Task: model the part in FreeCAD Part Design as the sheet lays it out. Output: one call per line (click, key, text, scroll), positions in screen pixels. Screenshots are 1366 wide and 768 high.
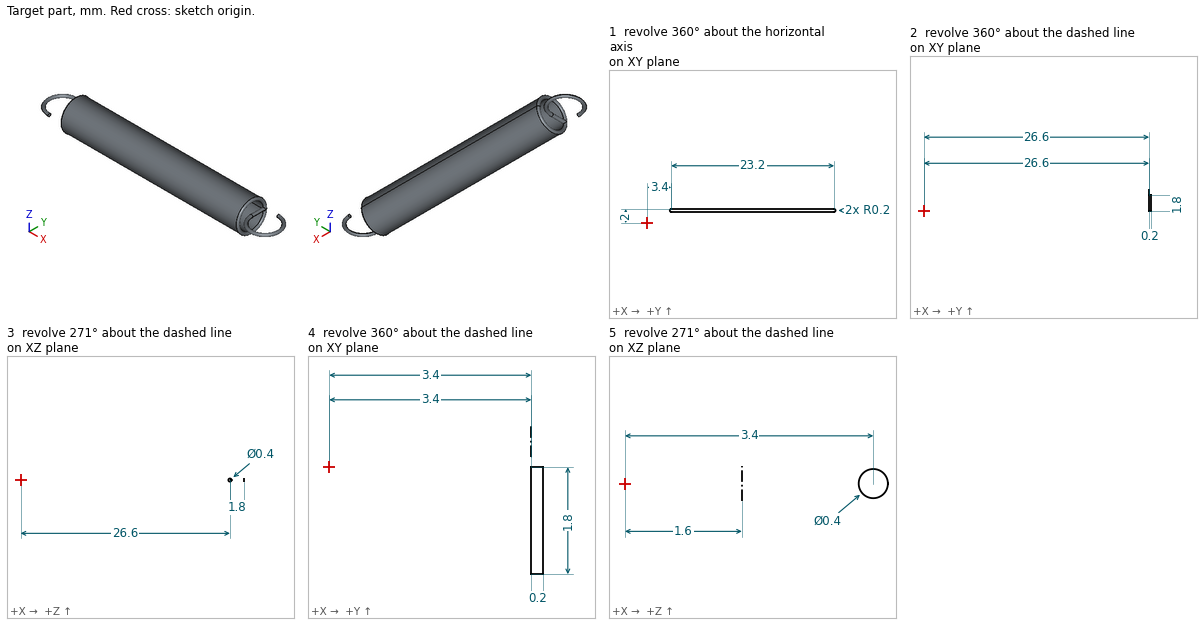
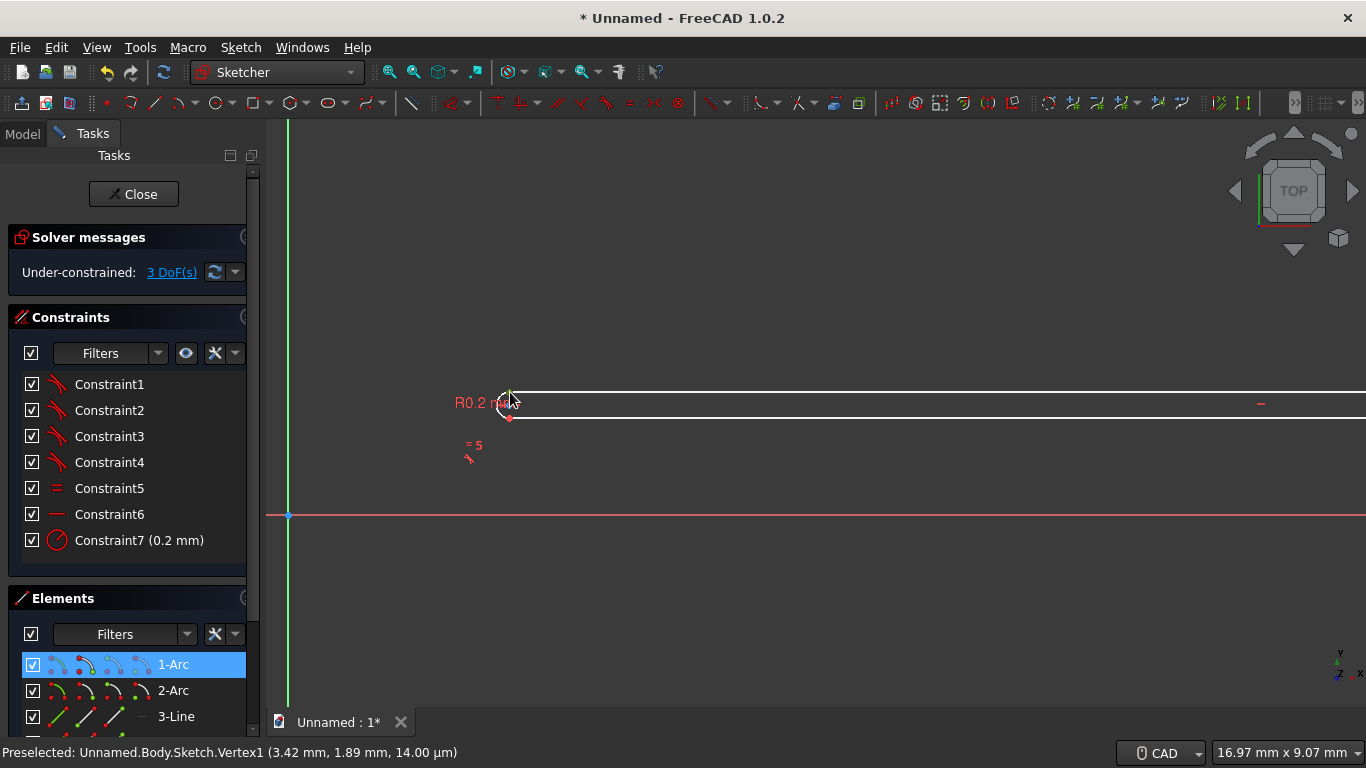
click(470, 104)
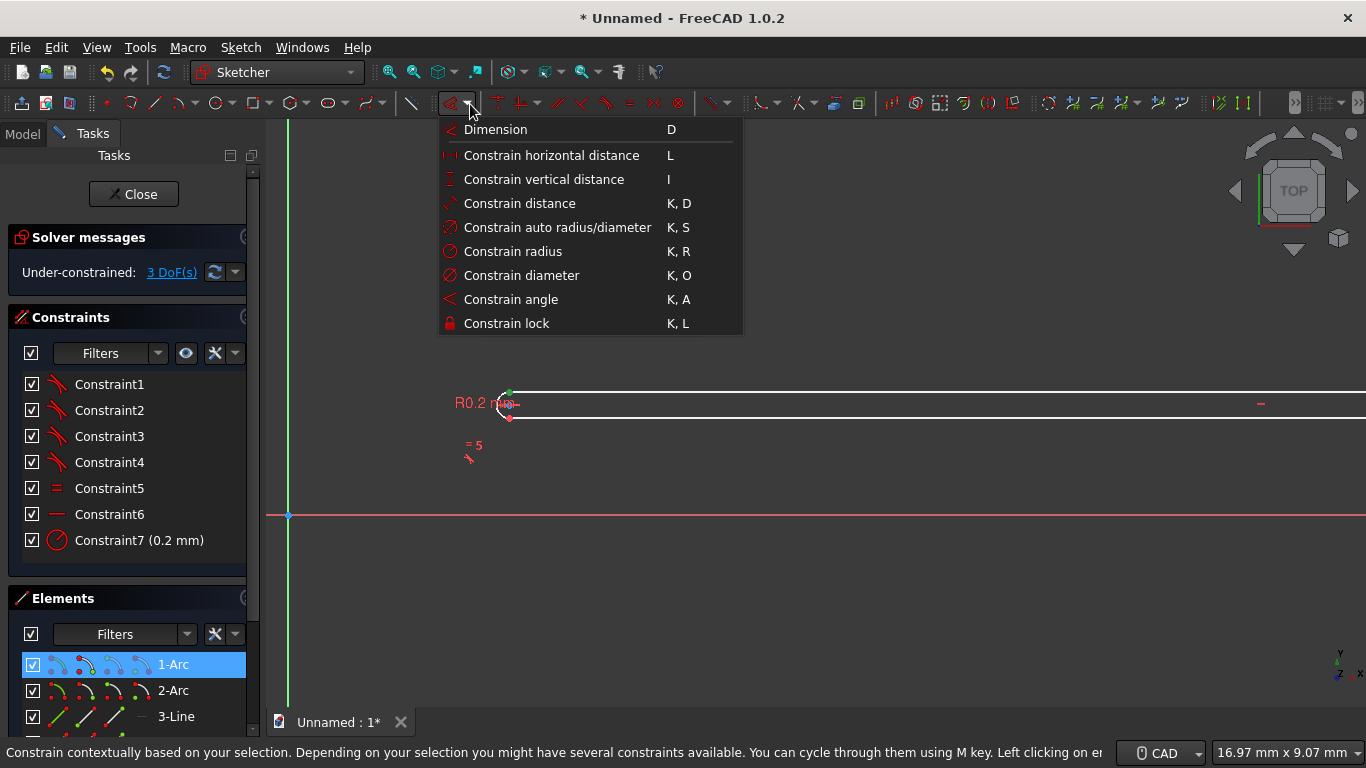
click(591, 179)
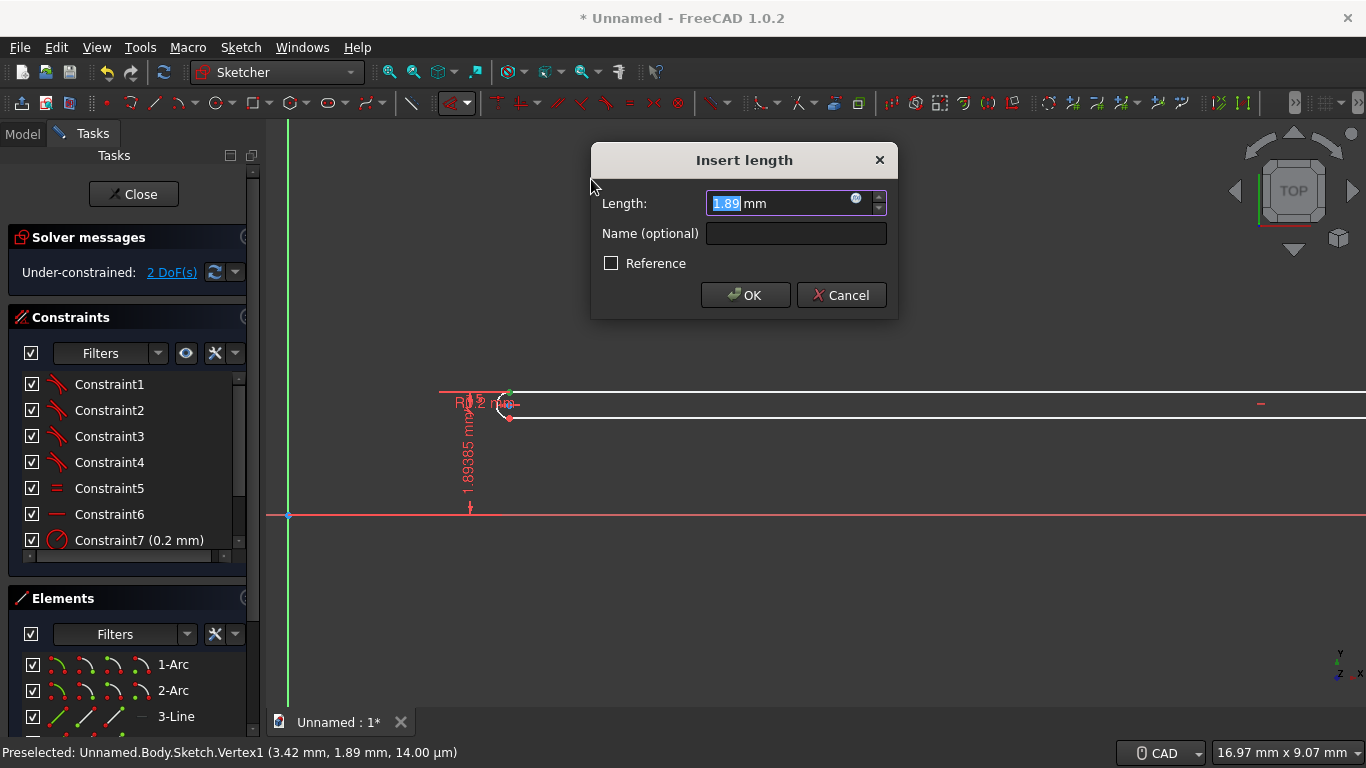
text(2)
key(Return)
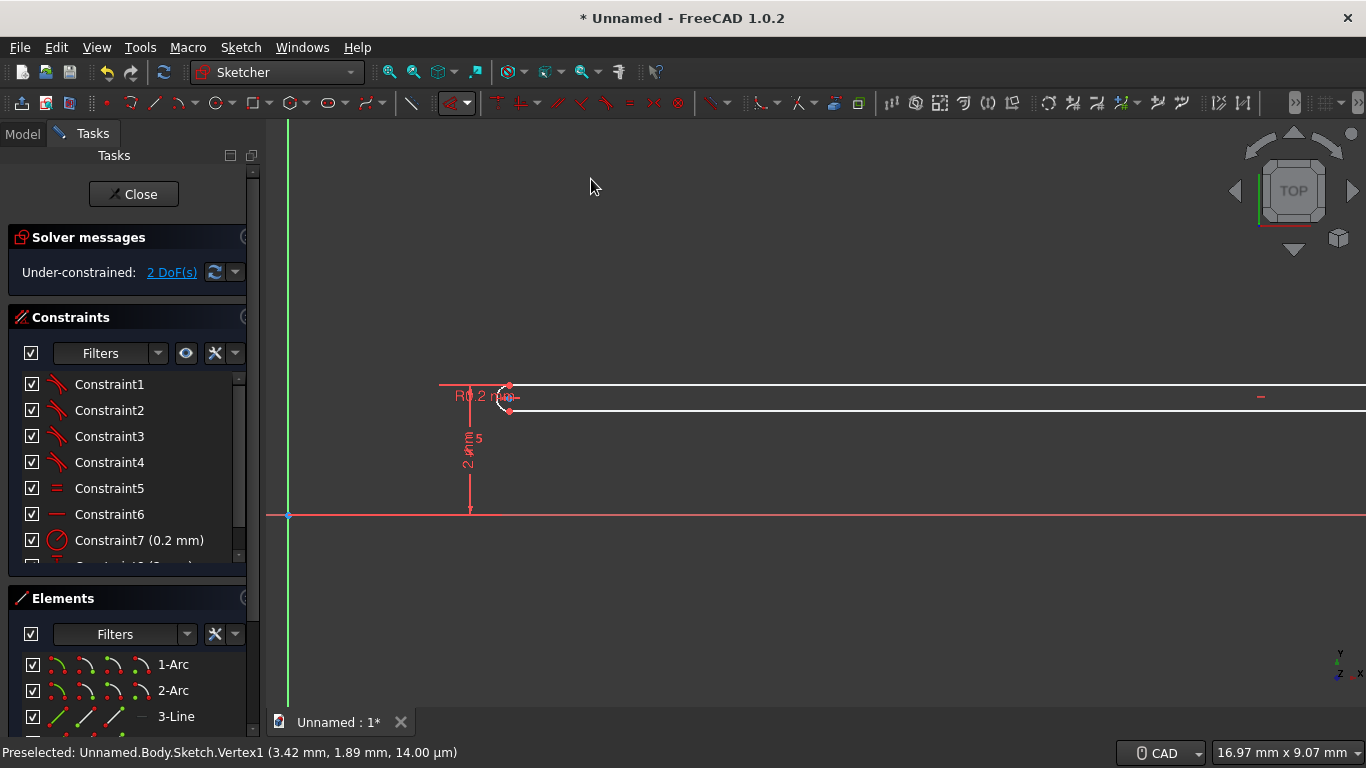
click(961, 385)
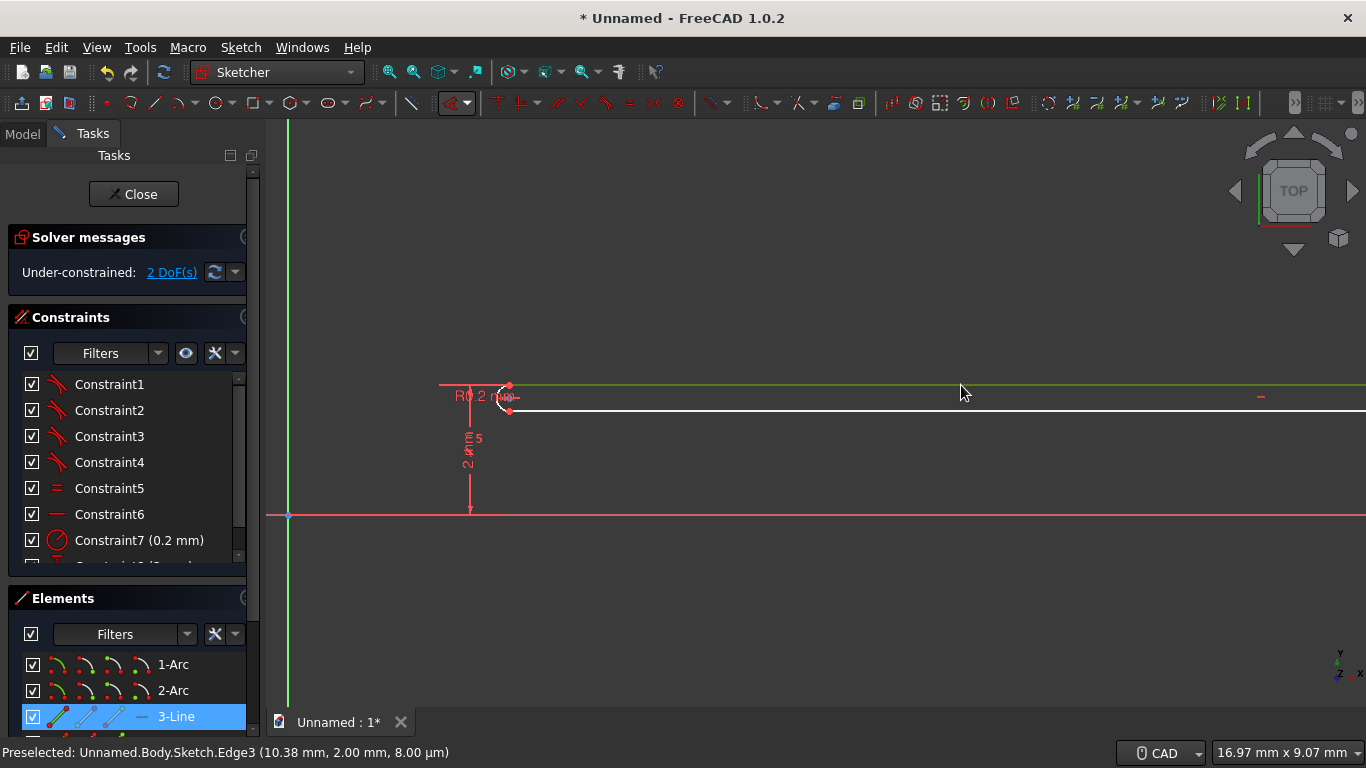
key(l)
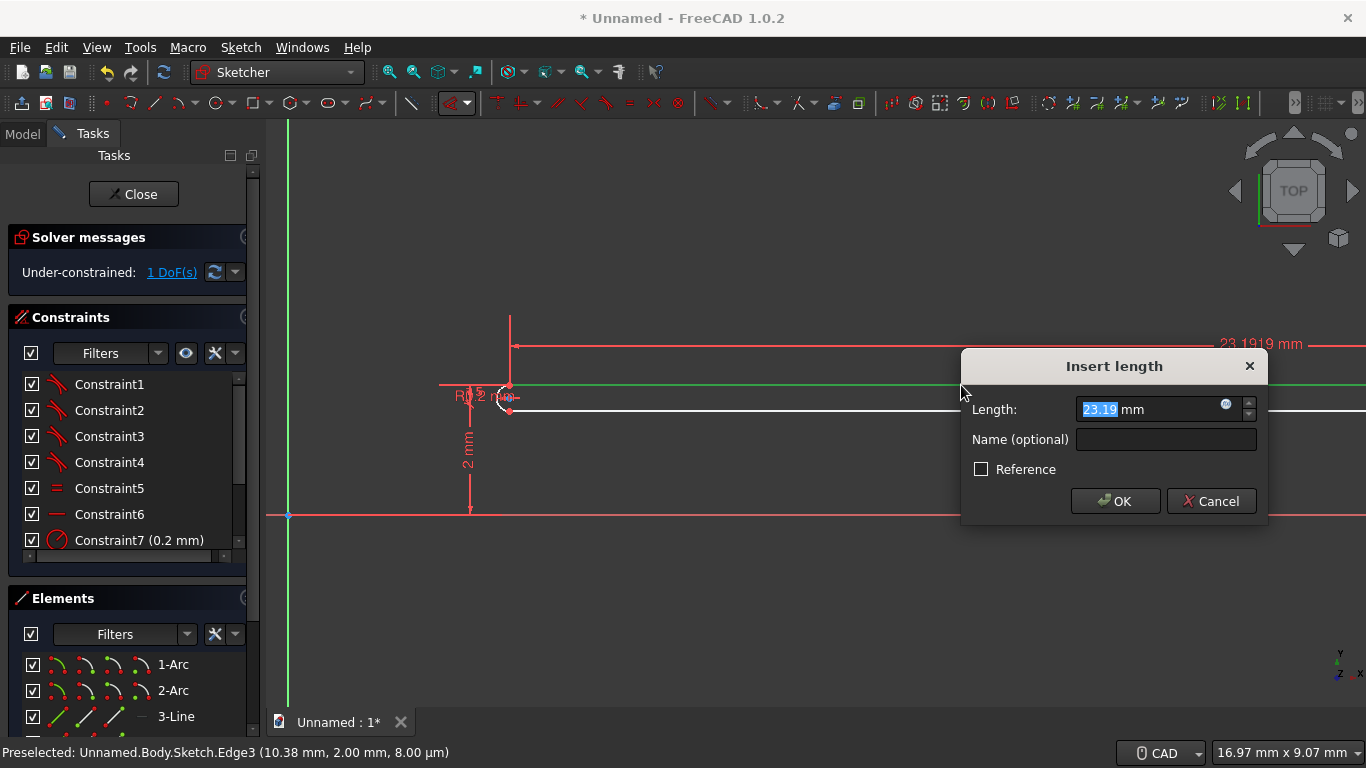
text(23.2)
key(Return)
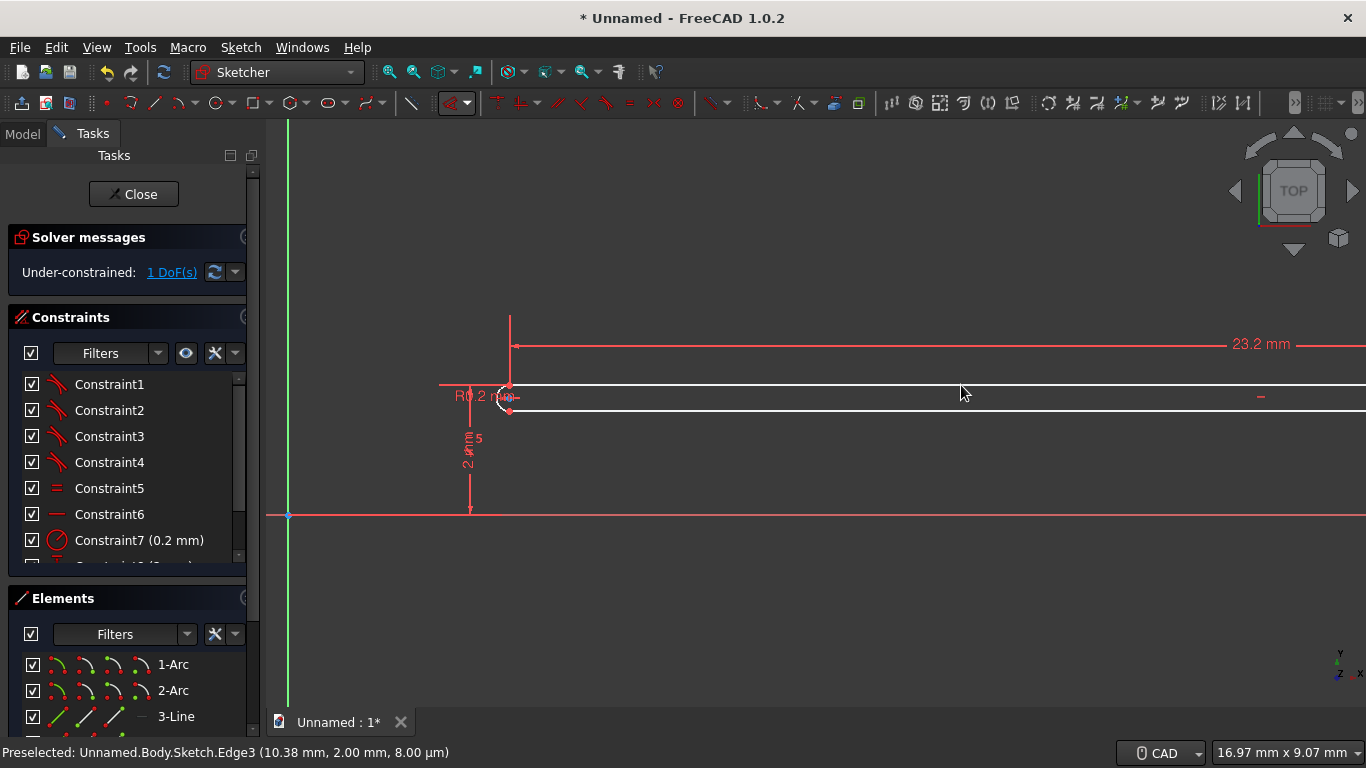
click(510, 385)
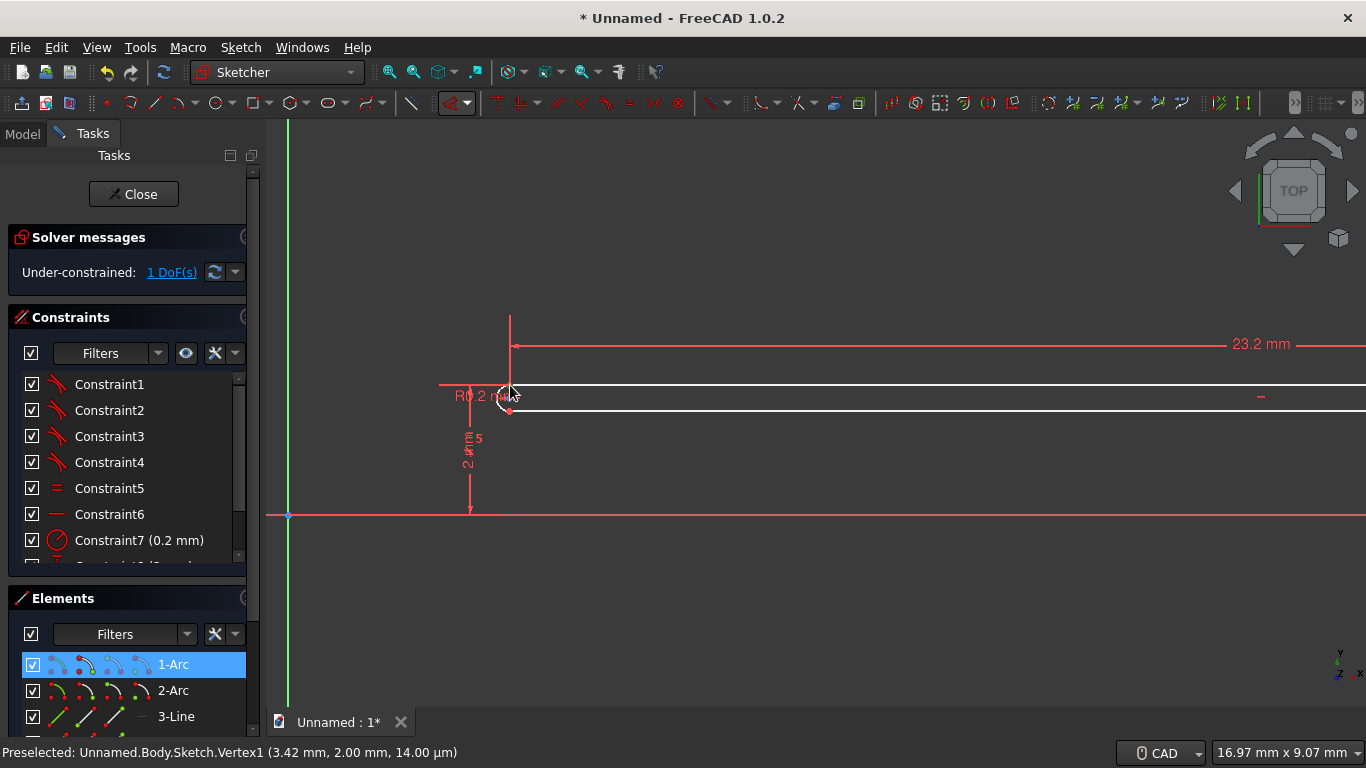
key(l)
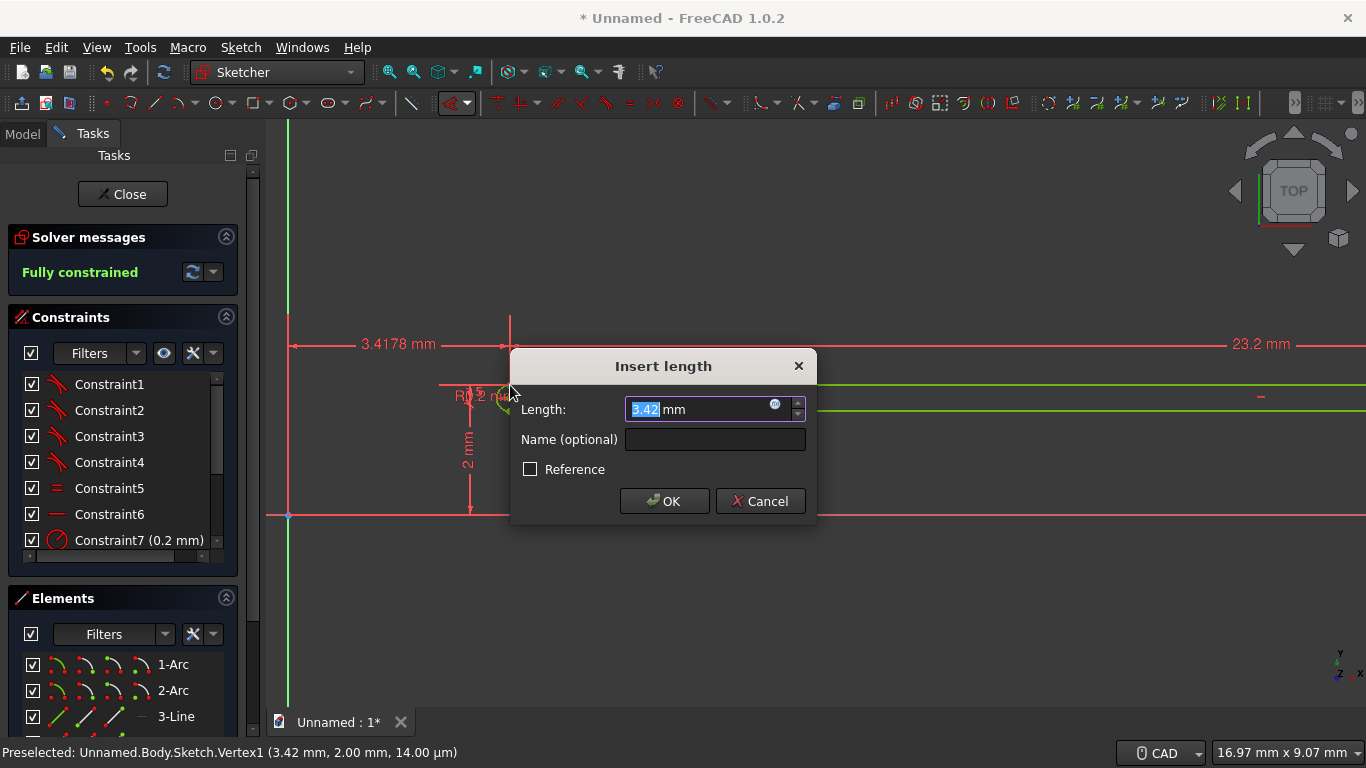
text(3.4)
key(Return)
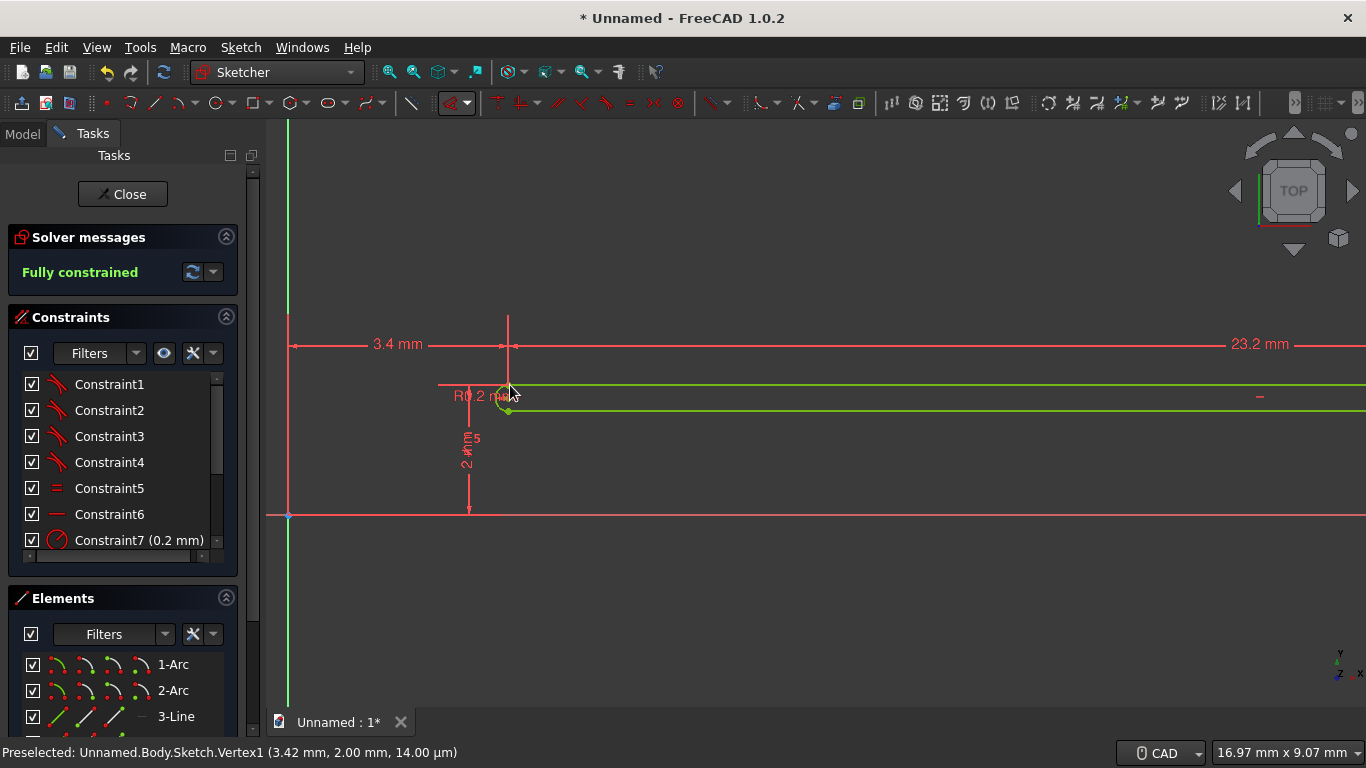
click(123, 194)